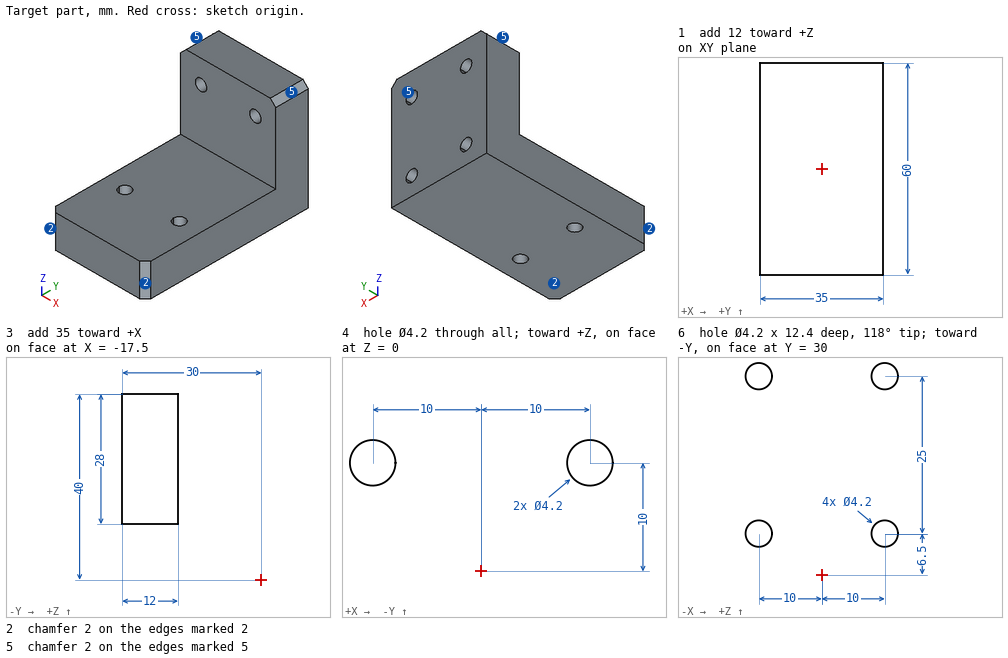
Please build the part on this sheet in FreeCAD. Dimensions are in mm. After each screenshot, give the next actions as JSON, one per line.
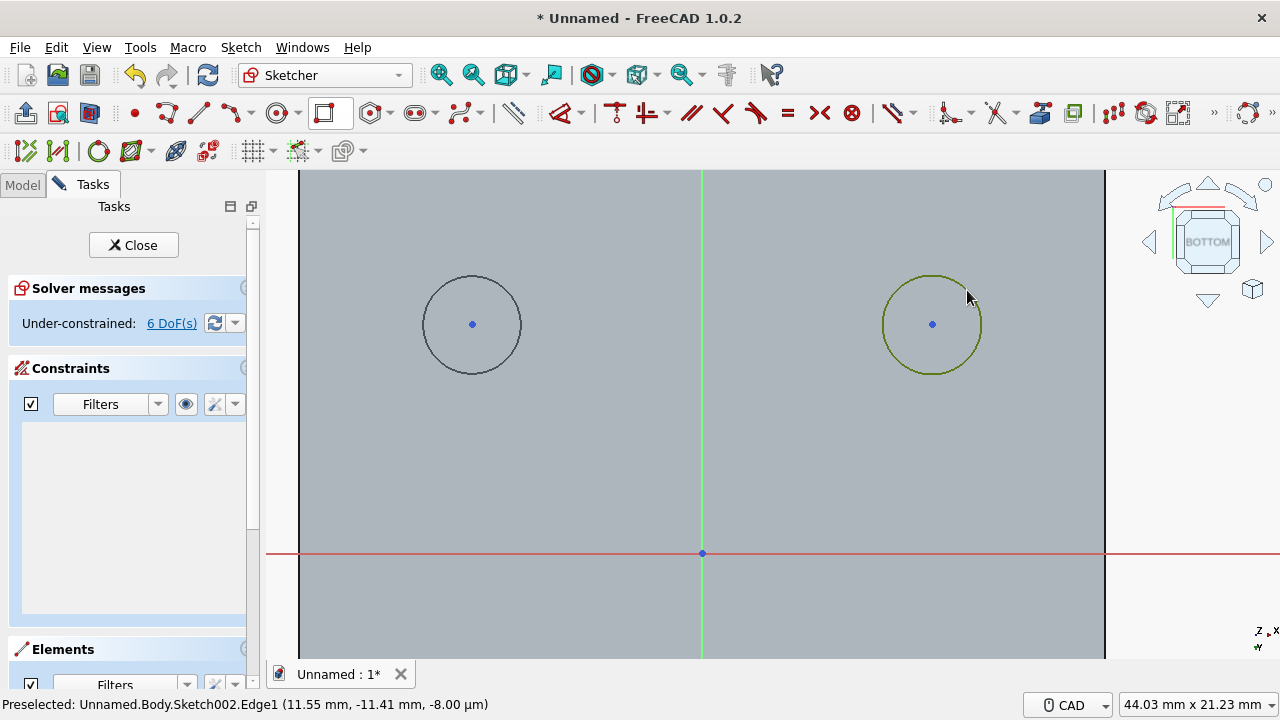
{"action": "left_click", "coordinate": [506, 290]}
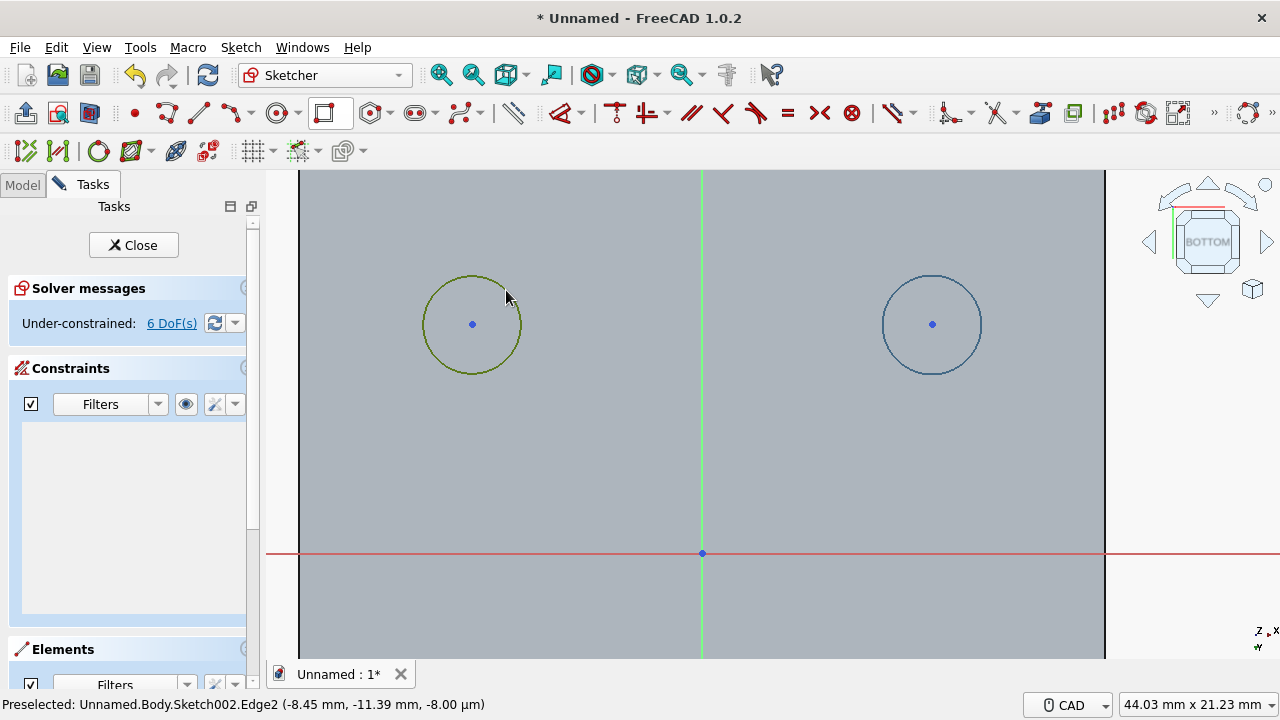
{"action": "left_click", "coordinate": [788, 114]}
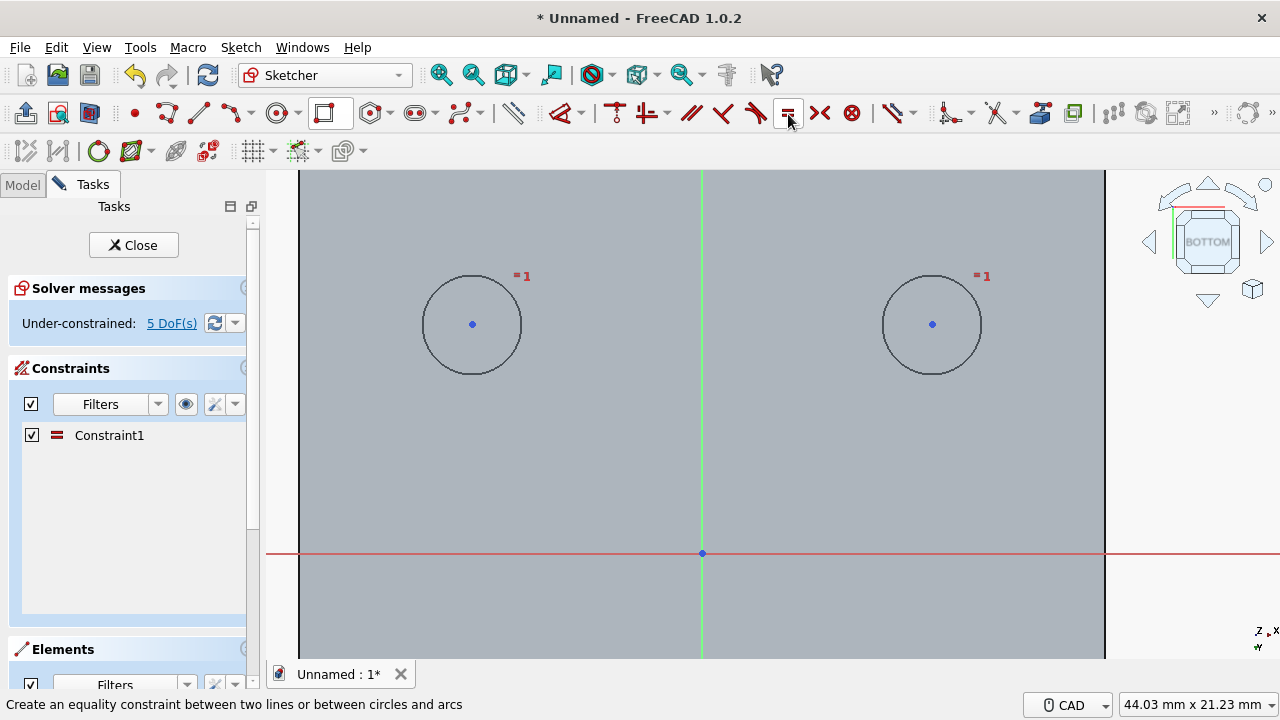
{"action": "left_click", "coordinate": [932, 325]}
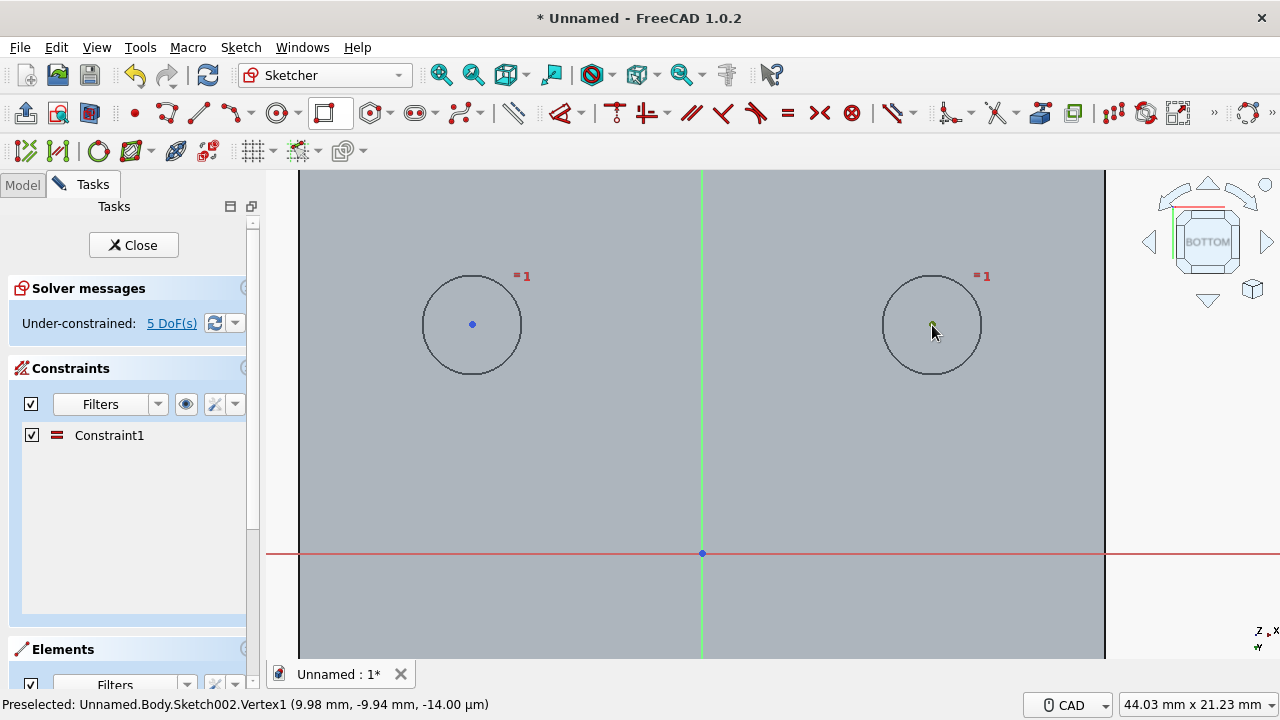
{"action": "left_click", "coordinate": [472, 325]}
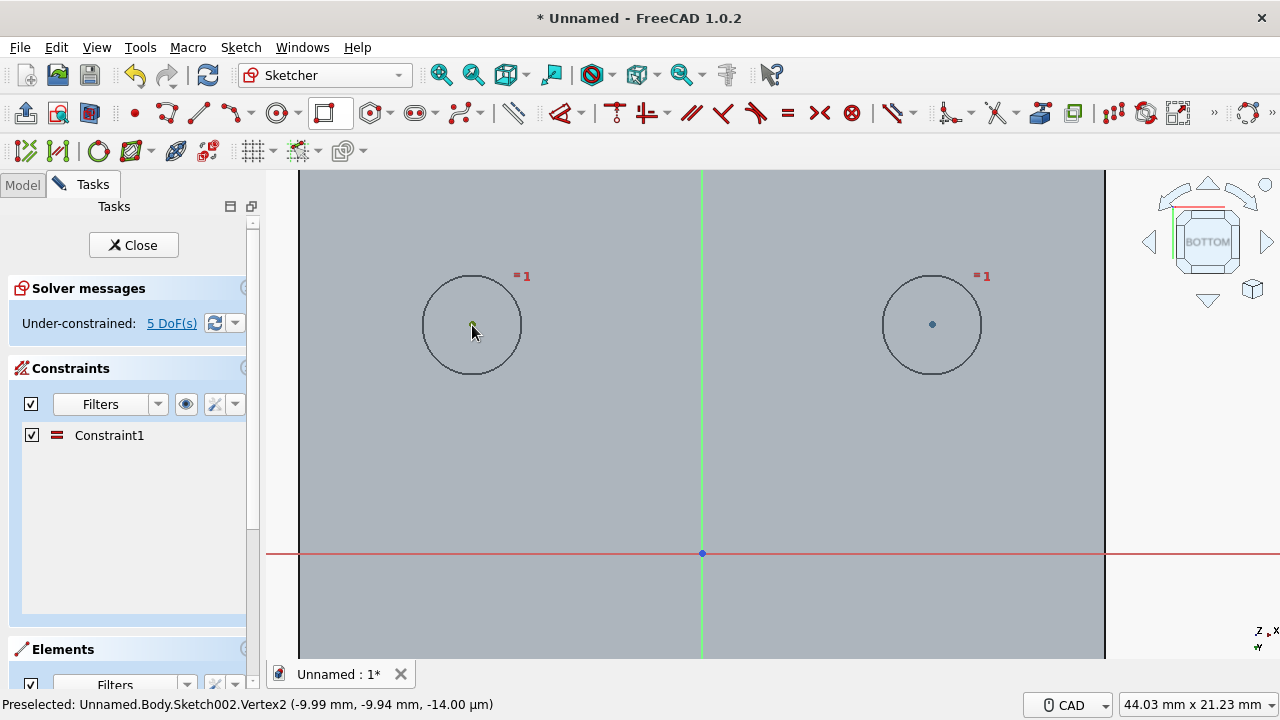
{"action": "key", "text": "h"}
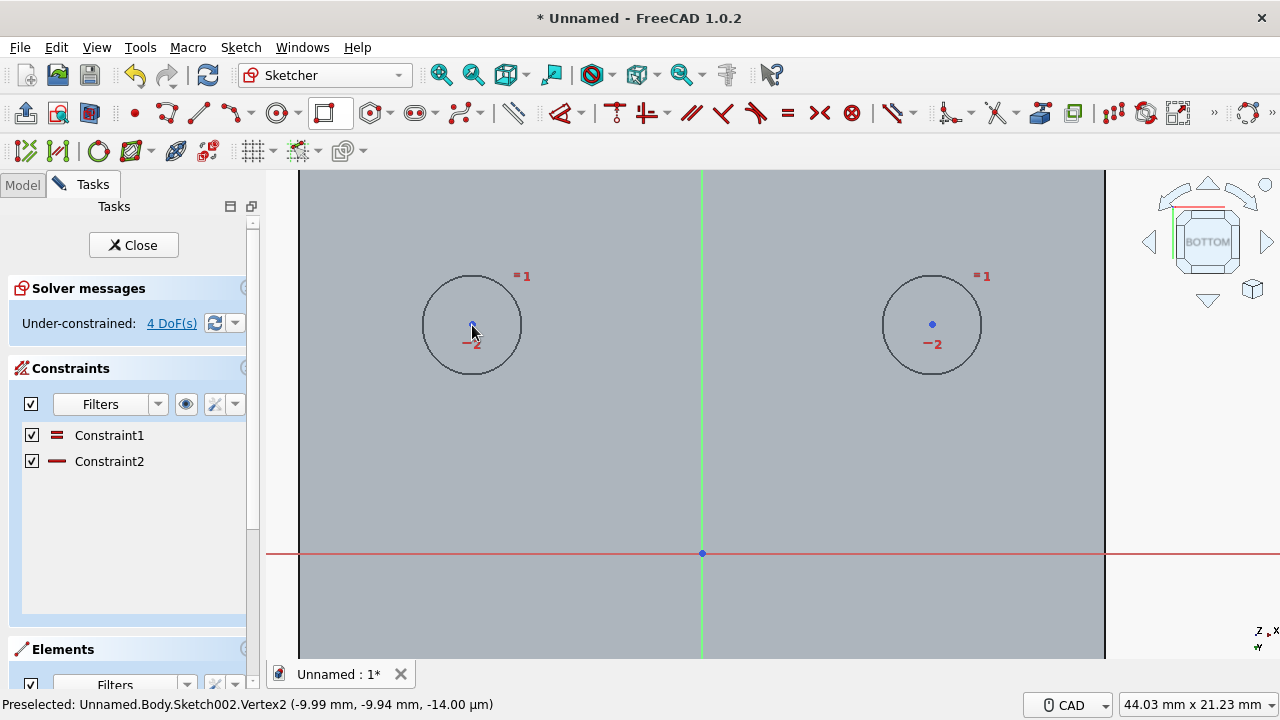
{"action": "left_click", "coordinate": [560, 114]}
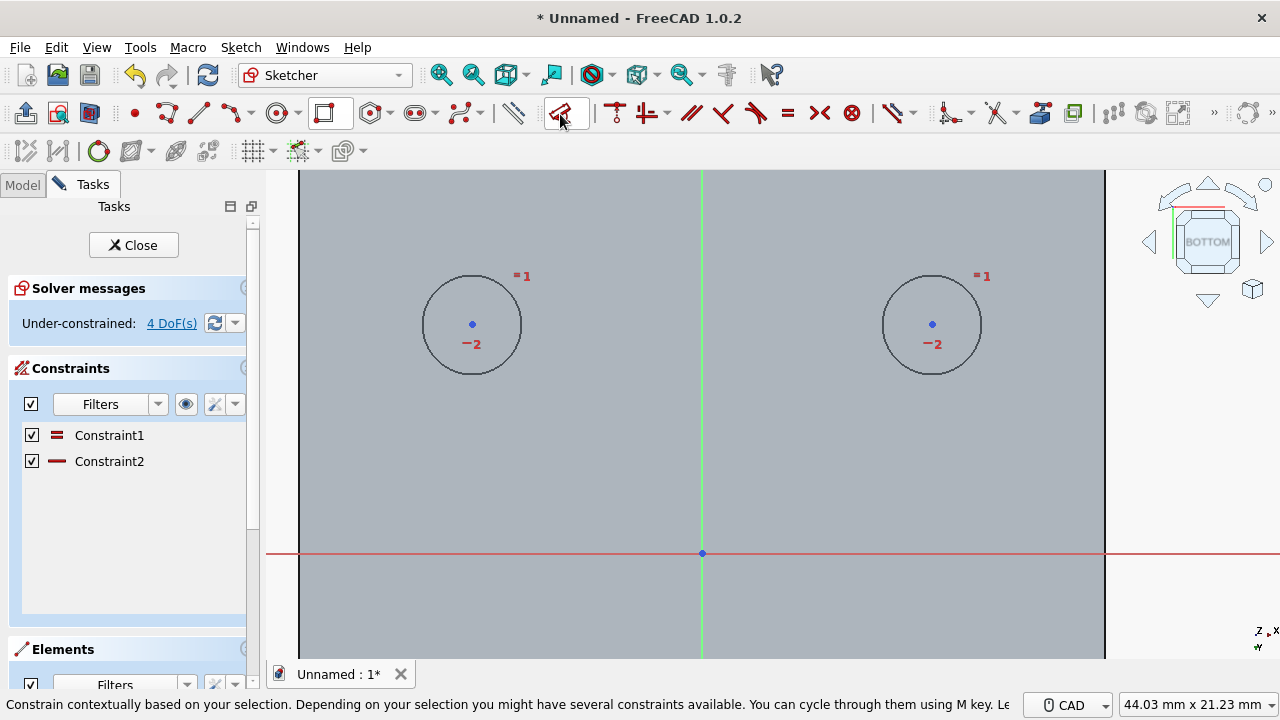
{"action": "left_click", "coordinate": [967, 290]}
{"action": "left_click", "coordinate": [990, 267]}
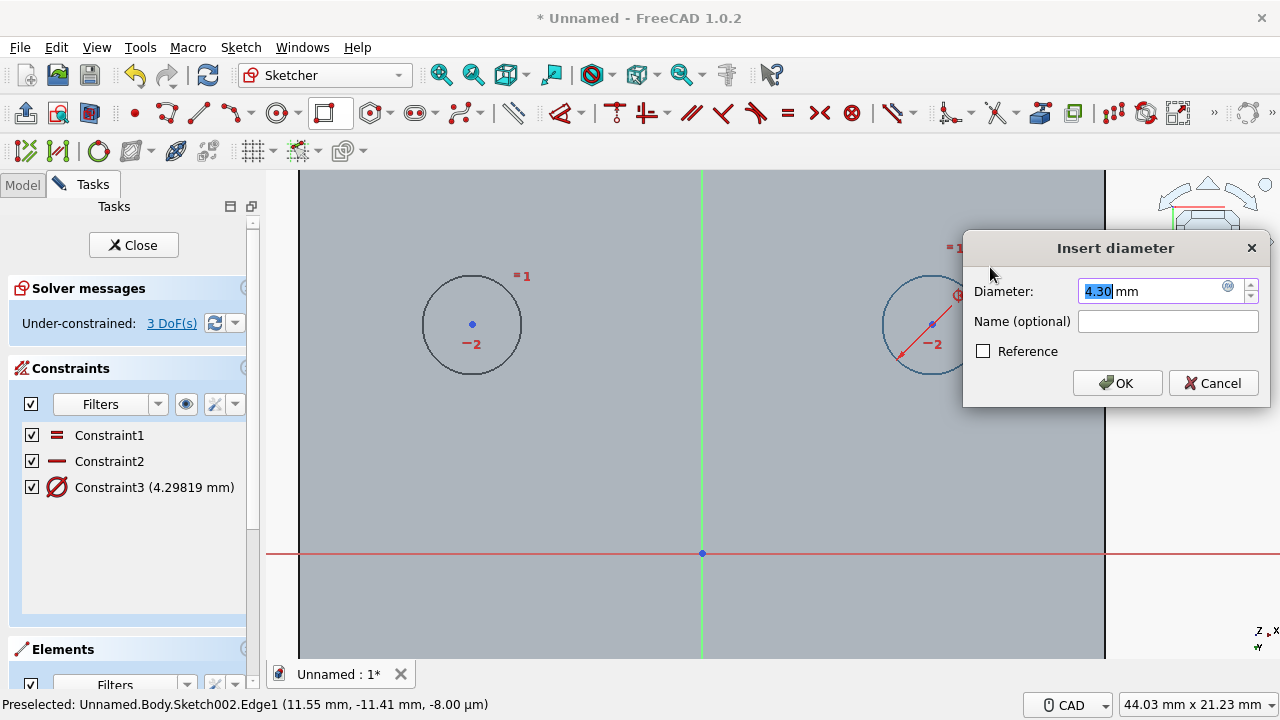
{"action": "type", "text": "4.2"}
{"action": "key", "text": "Return"}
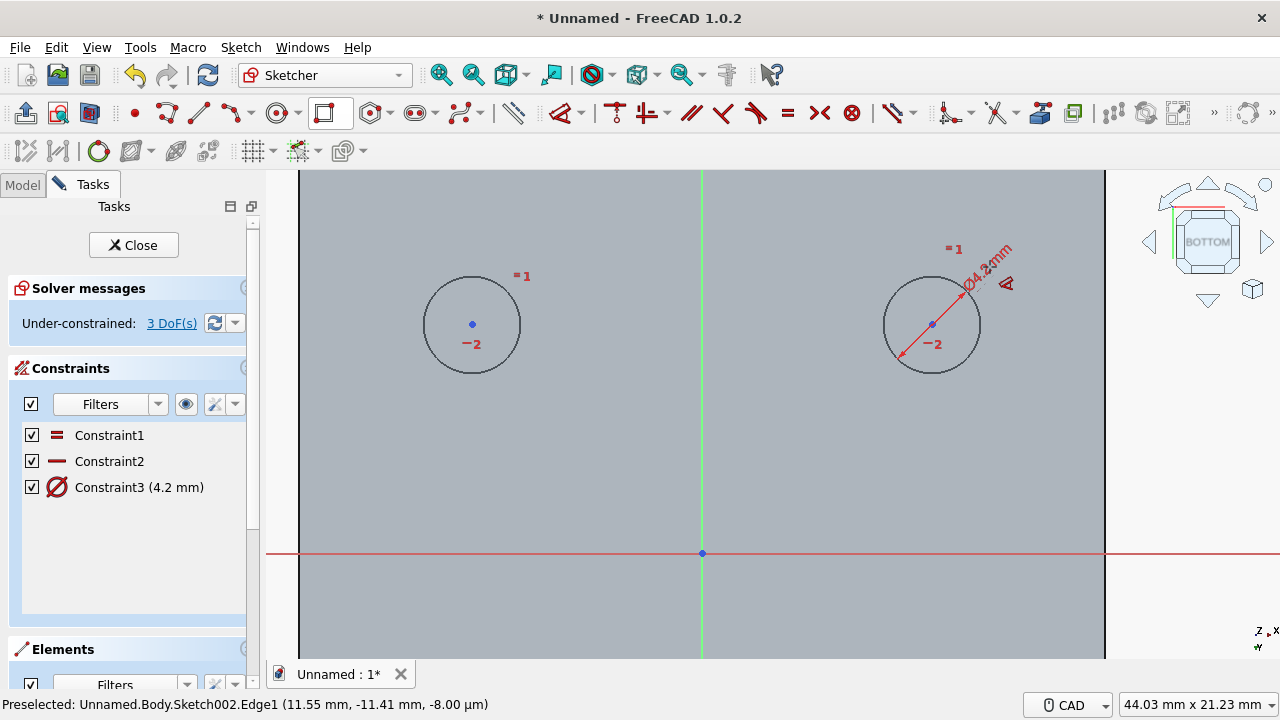
{"action": "left_click", "coordinate": [932, 325]}
{"action": "left_click", "coordinate": [817, 588]}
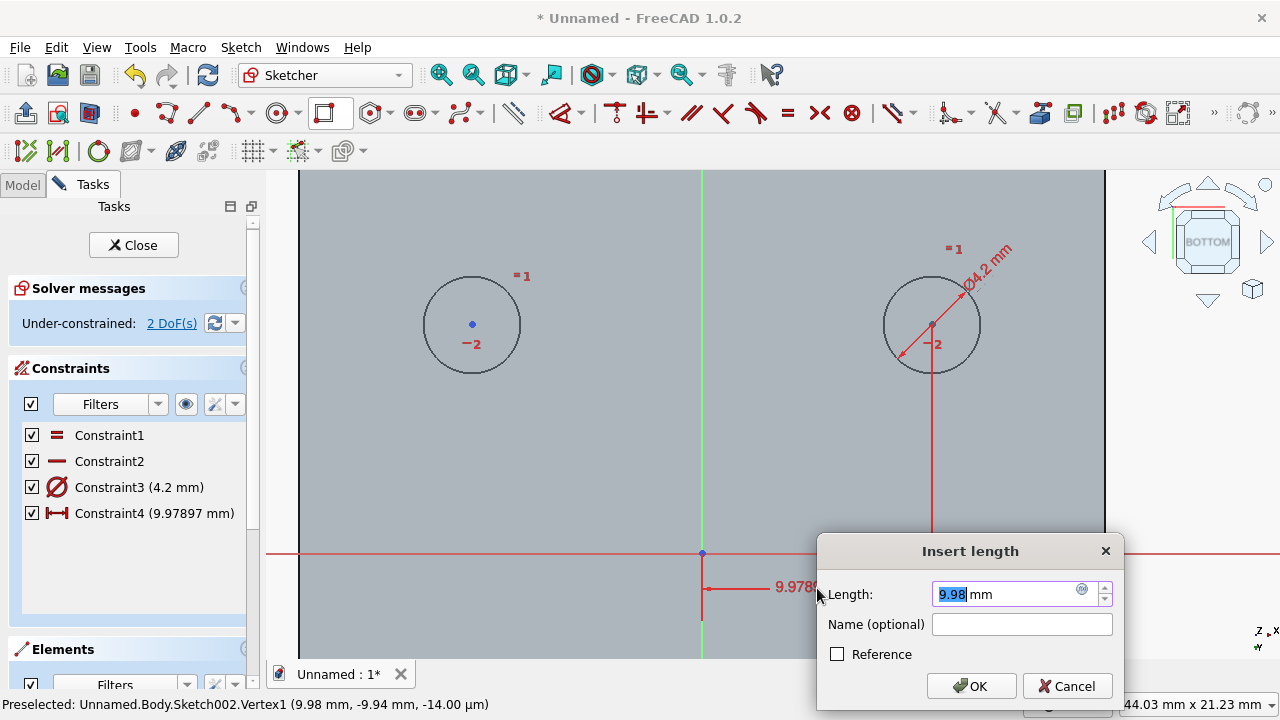
{"action": "type", "text": "10"}
{"action": "key", "text": "Return"}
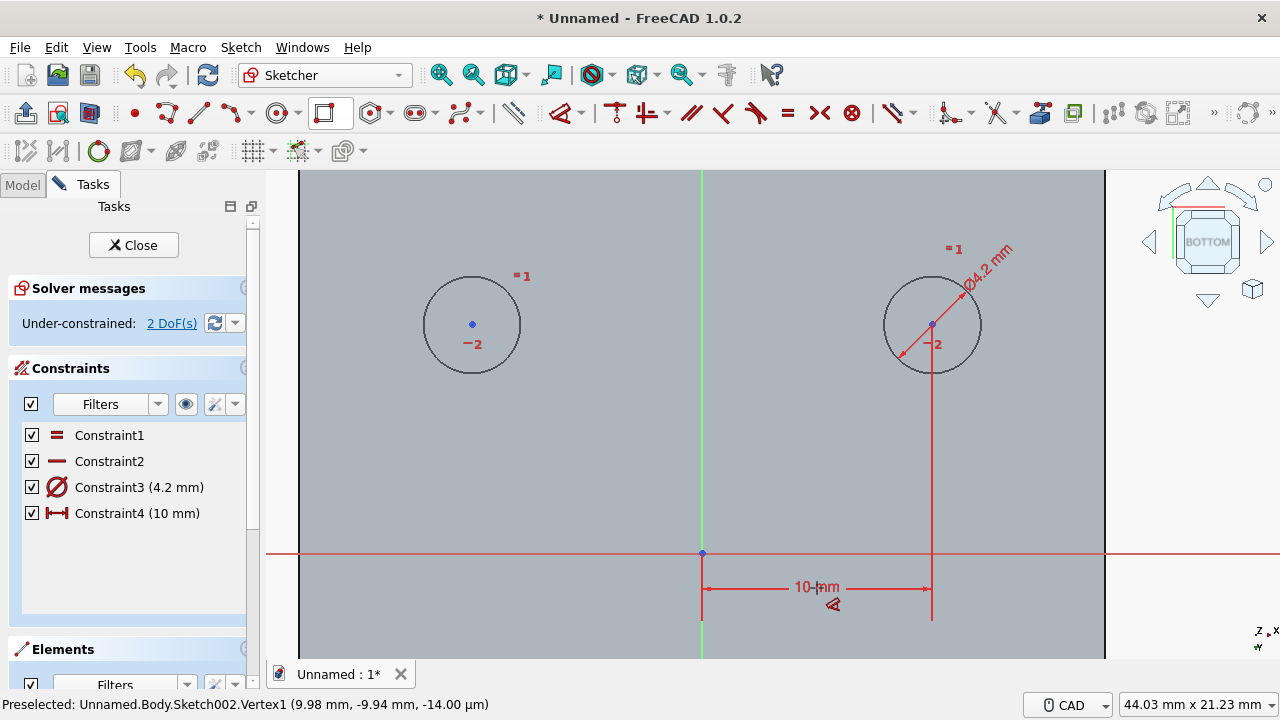
{"action": "left_click", "coordinate": [932, 325]}
{"action": "left_click", "coordinate": [966, 439]}